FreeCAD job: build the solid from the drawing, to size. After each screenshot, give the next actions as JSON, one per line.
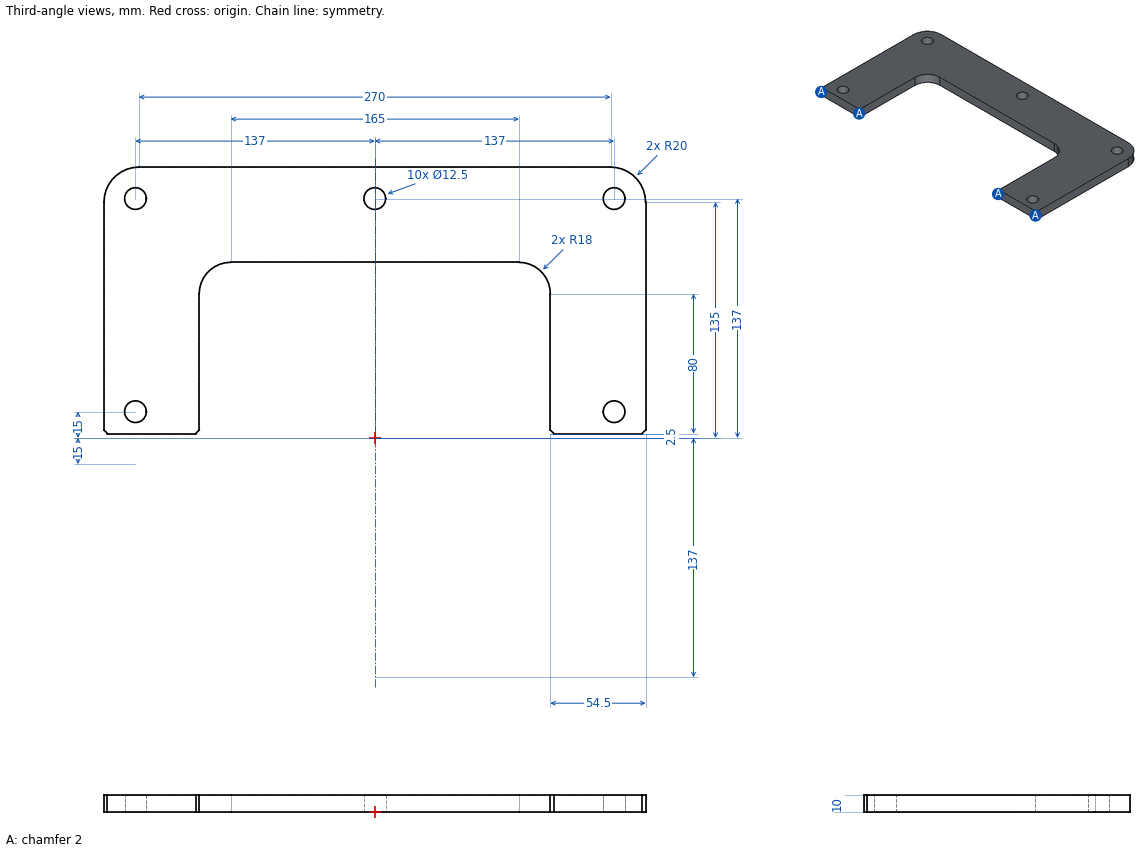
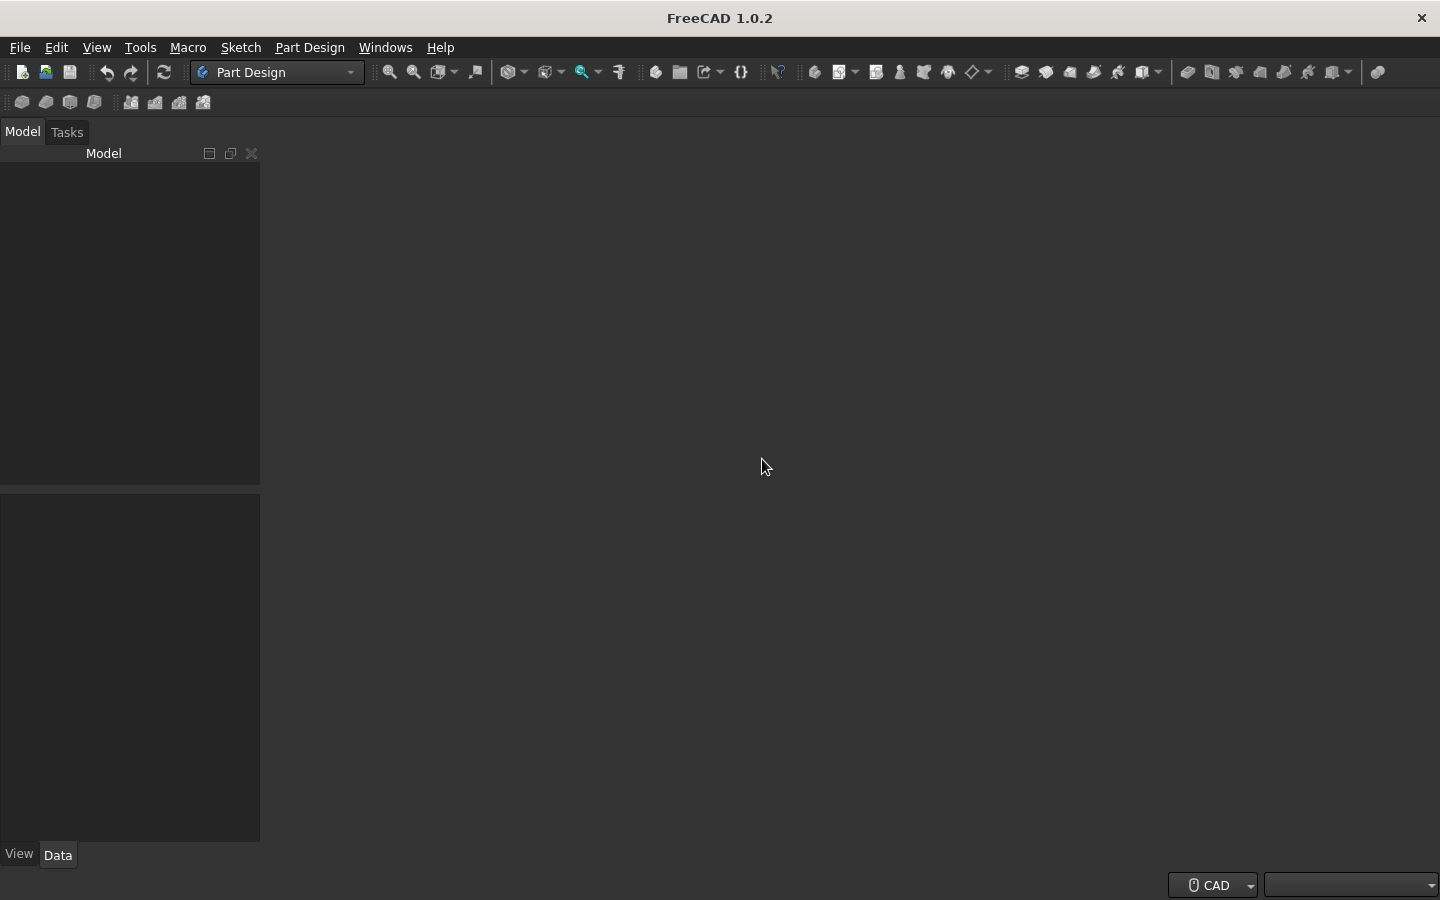
{"action": "key", "text": "ctrl+n"}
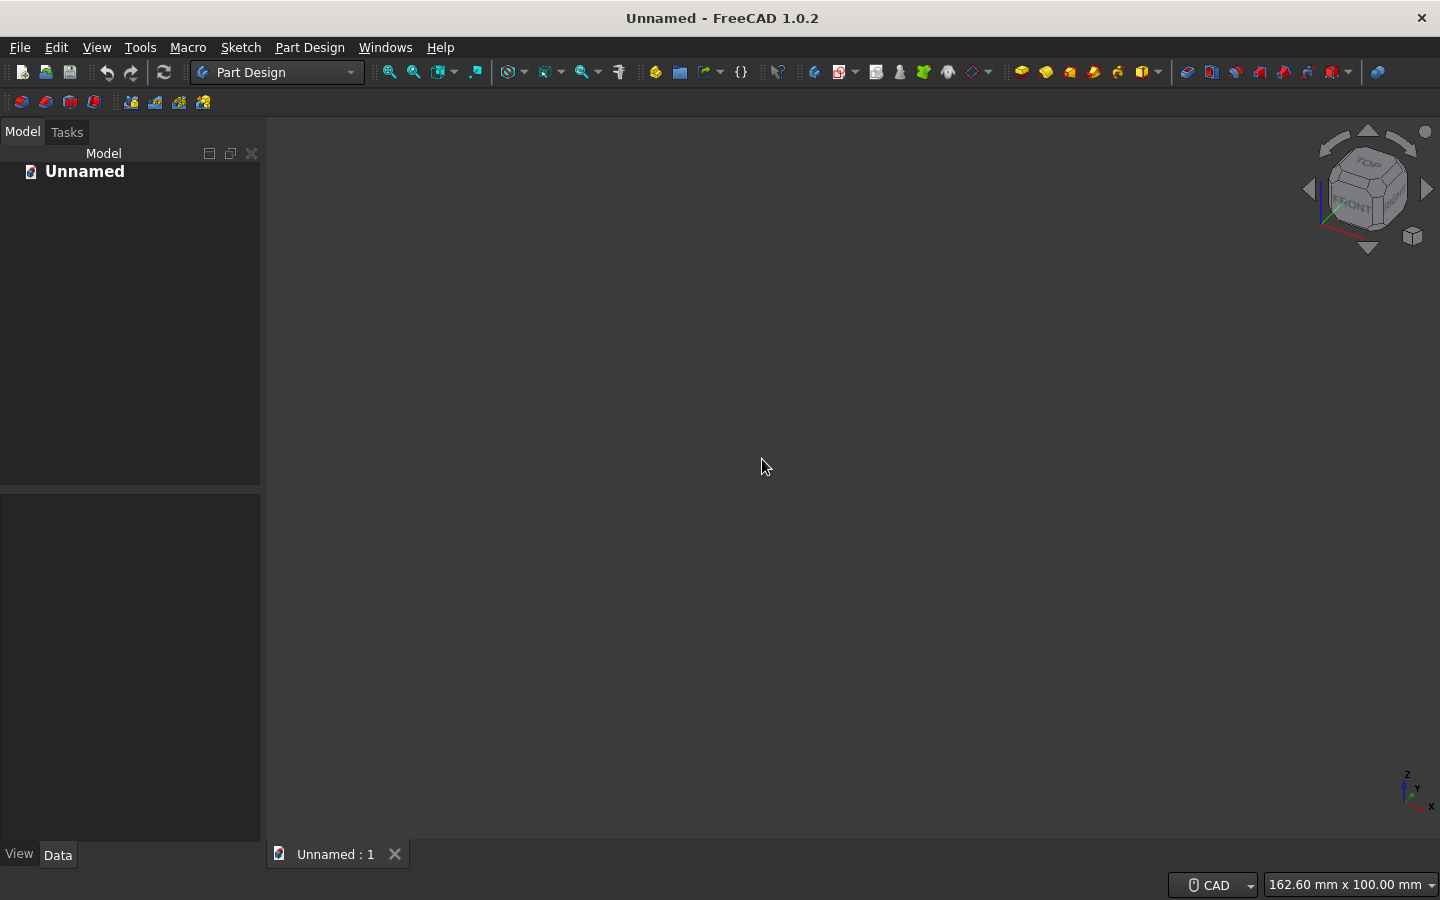
{"action": "left_click", "coordinate": [840, 72]}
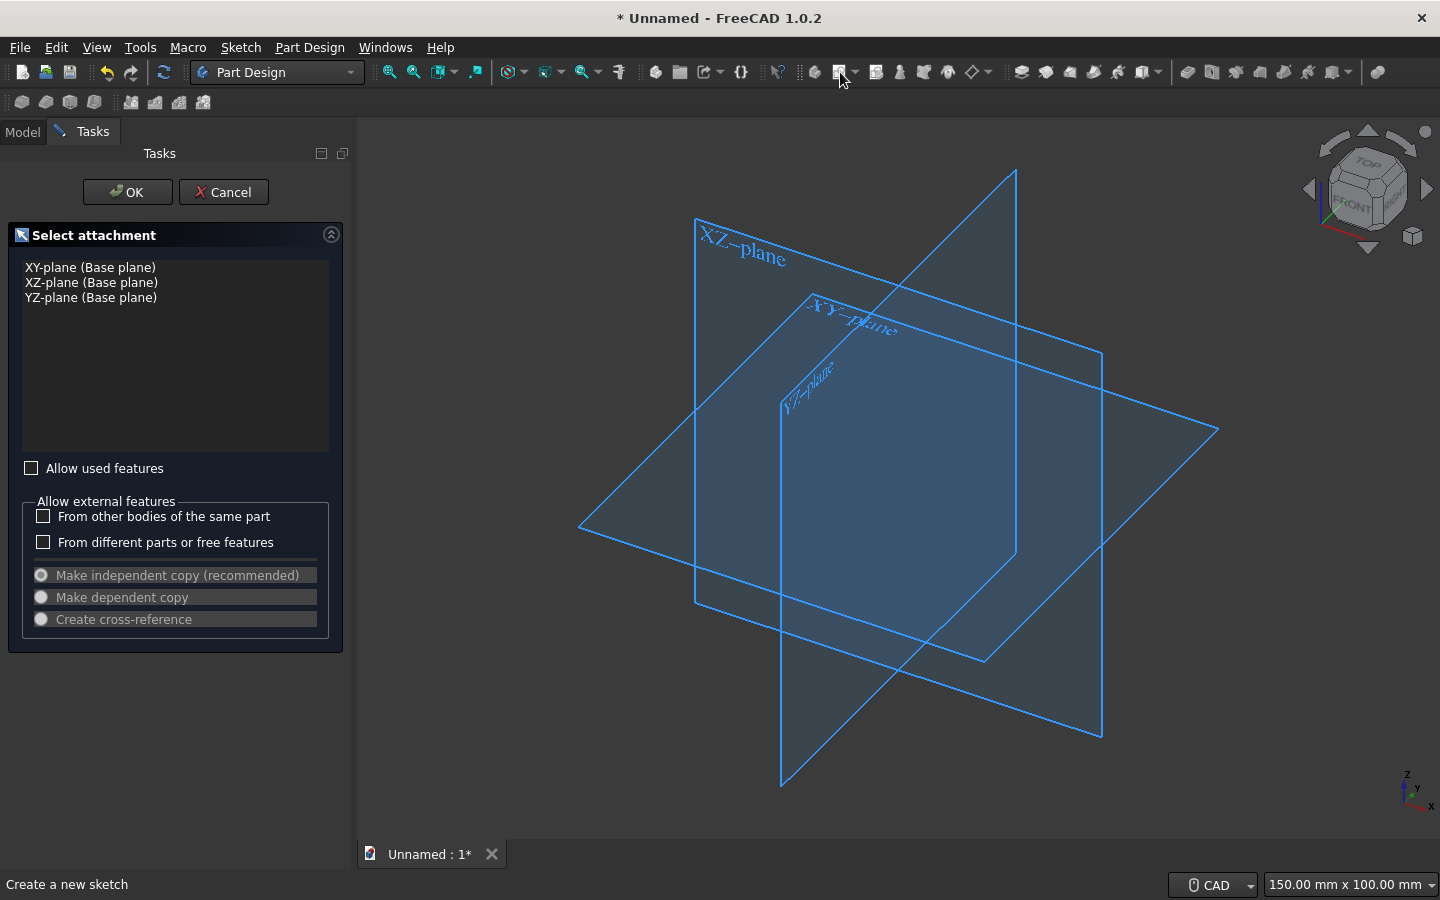
{"action": "left_click", "coordinate": [82, 268]}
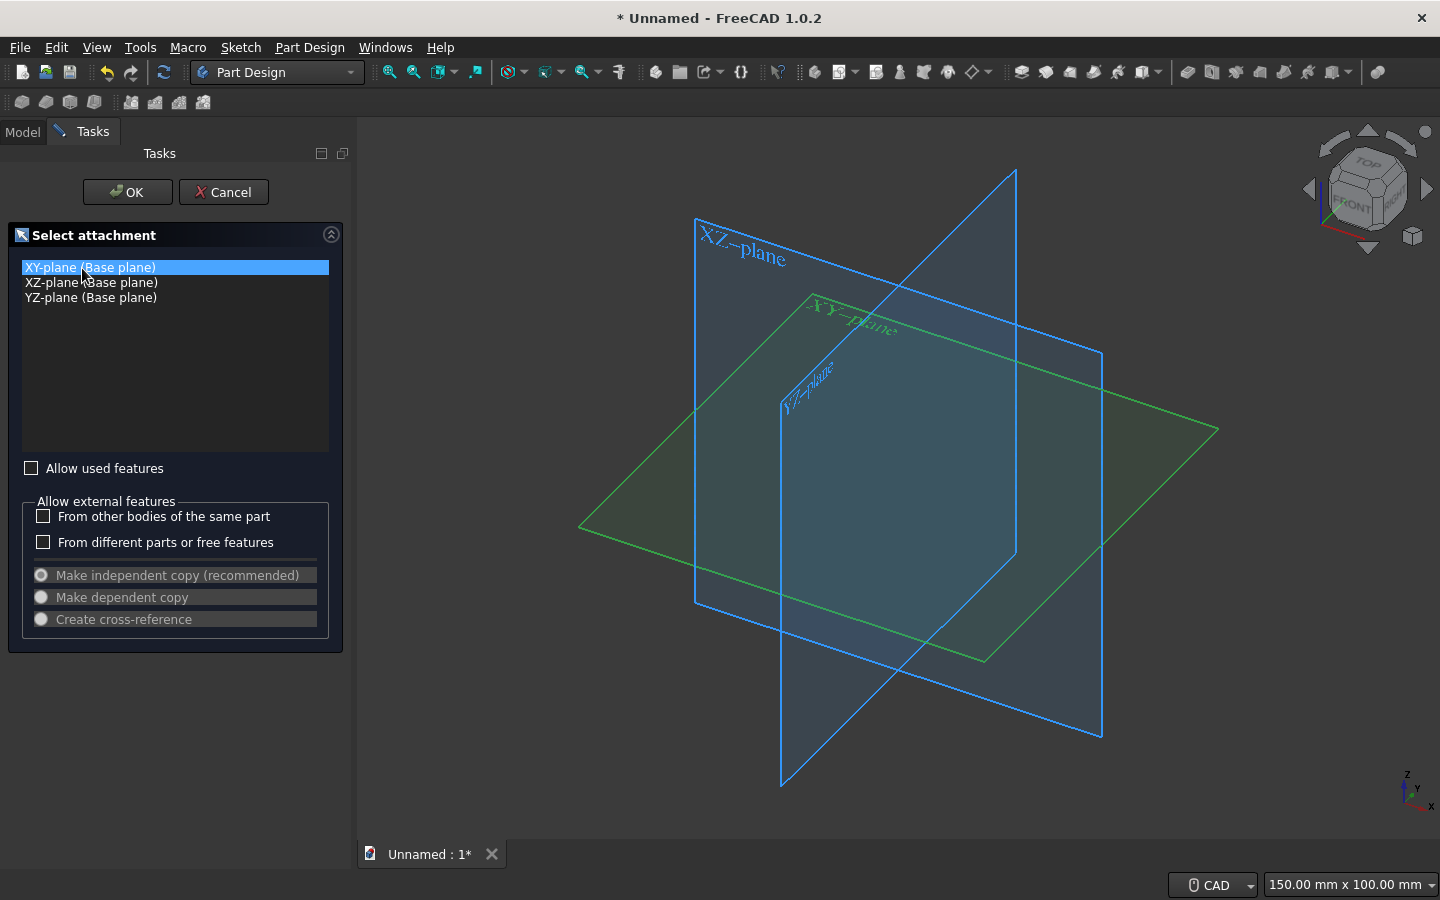
{"action": "left_click", "coordinate": [128, 192]}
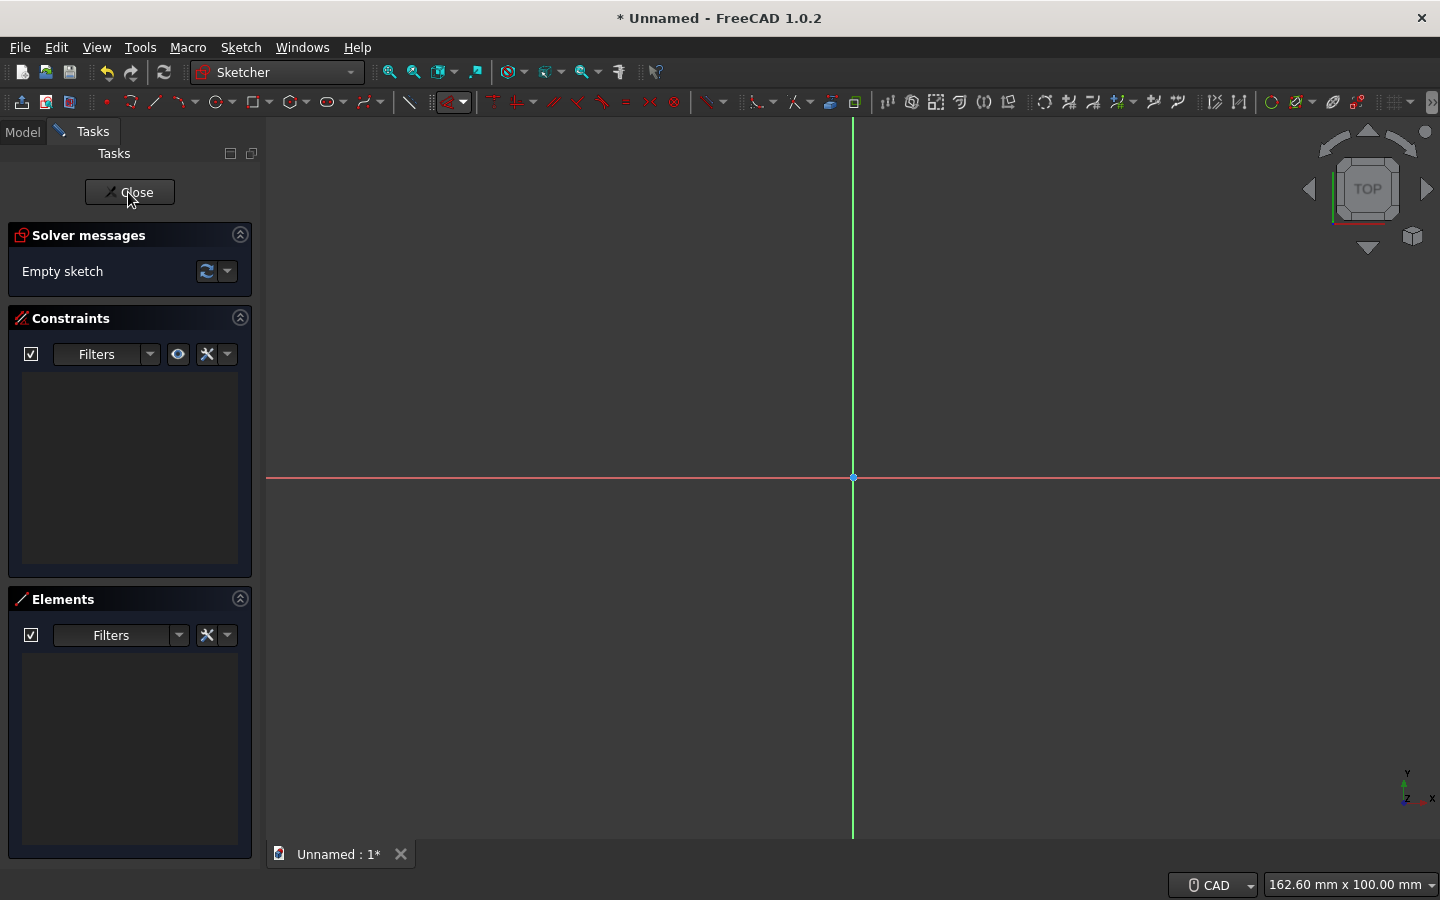
{"action": "scroll", "coordinate": [755, 719], "scroll_direction": "down", "scroll_amount": 6}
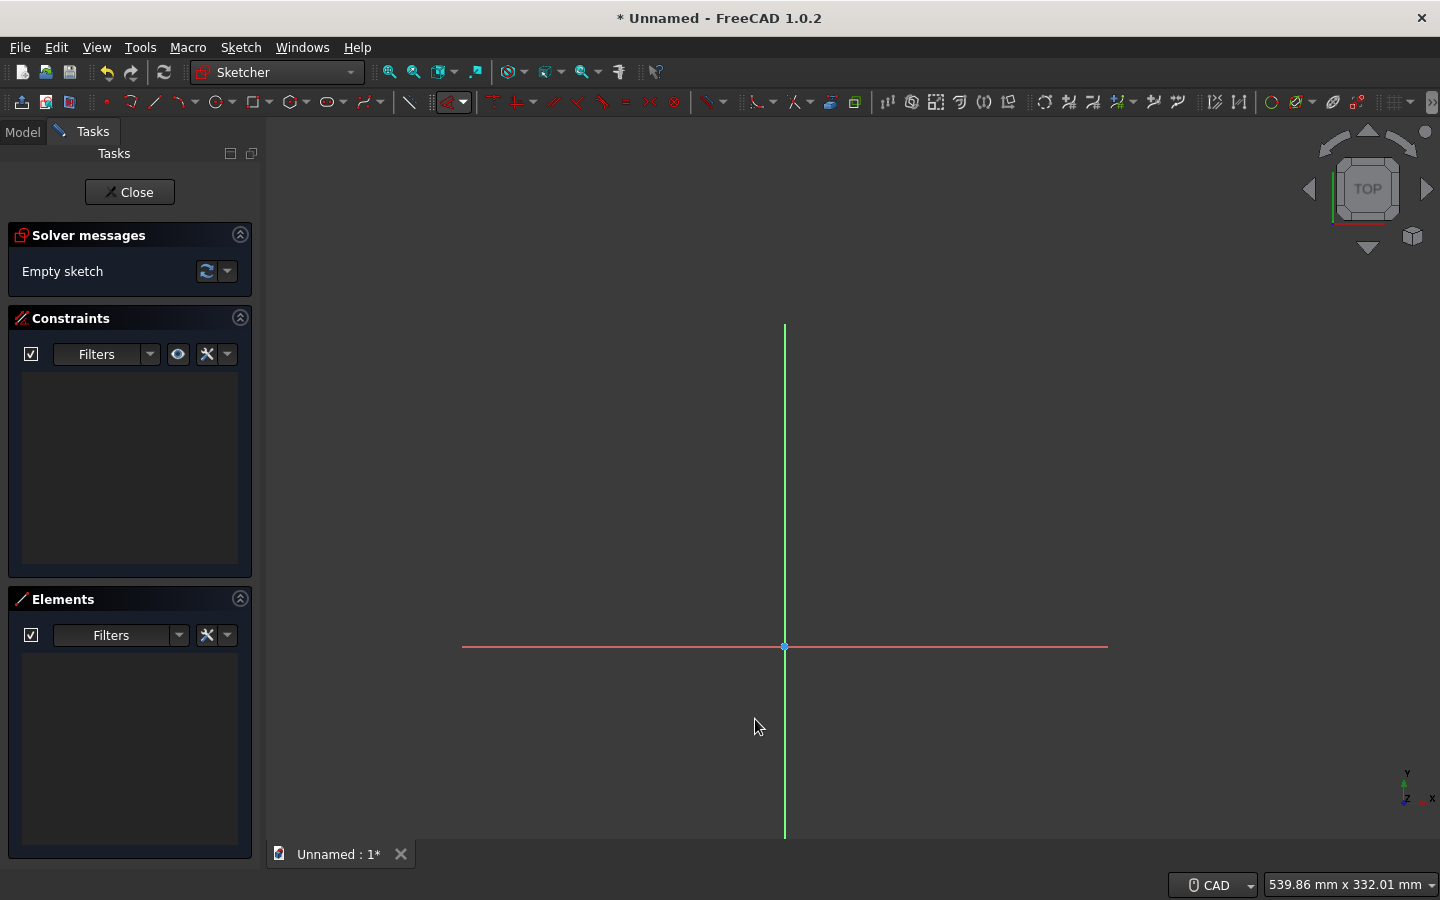
{"action": "key", "text": "g l"}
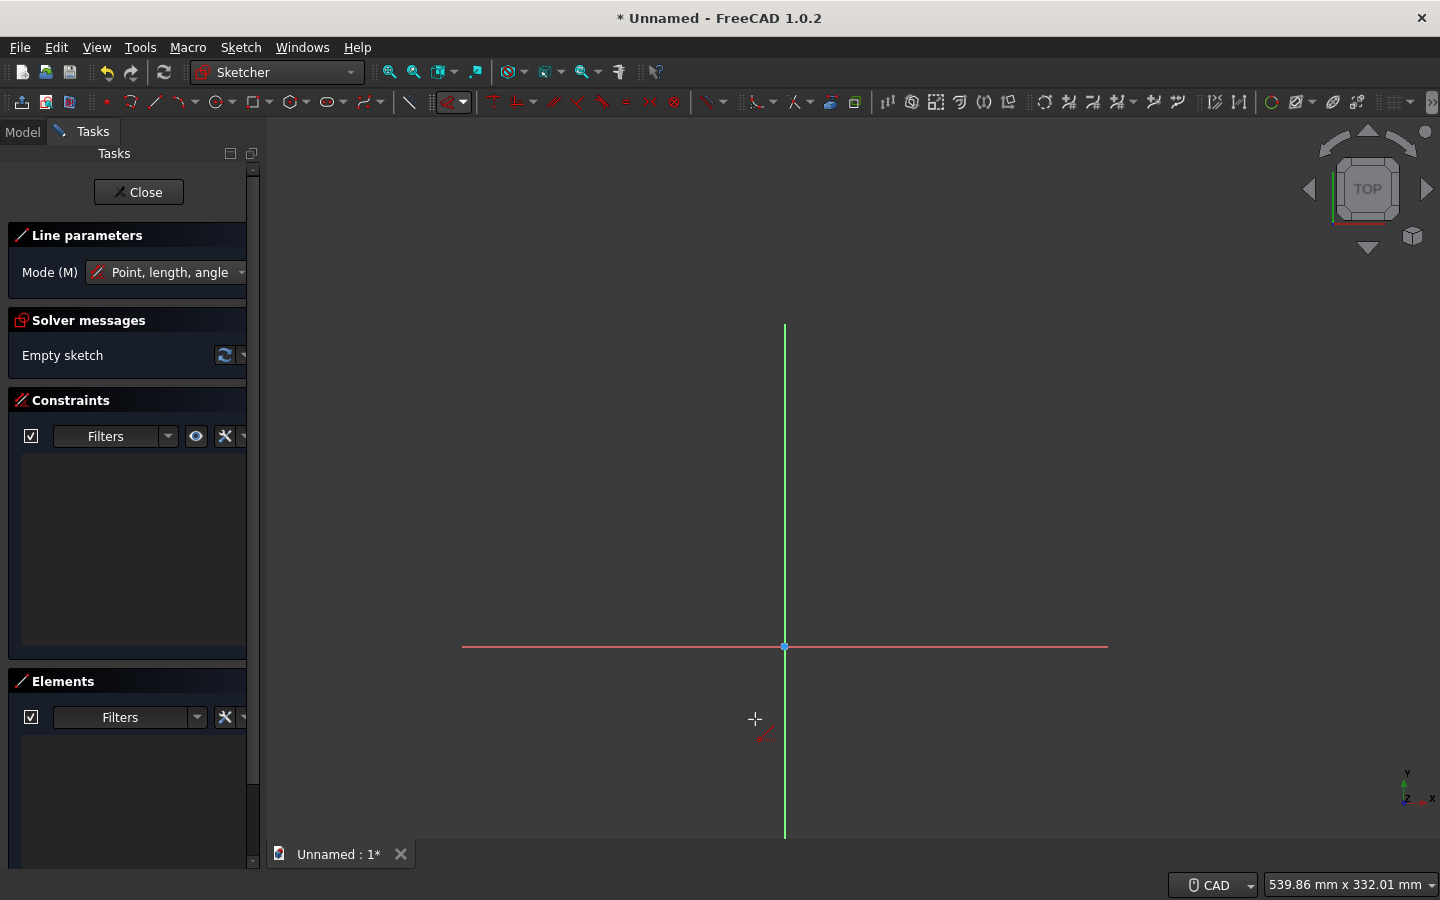
{"action": "left_click", "coordinate": [605, 428]}
{"action": "left_click", "coordinate": [964, 428]}